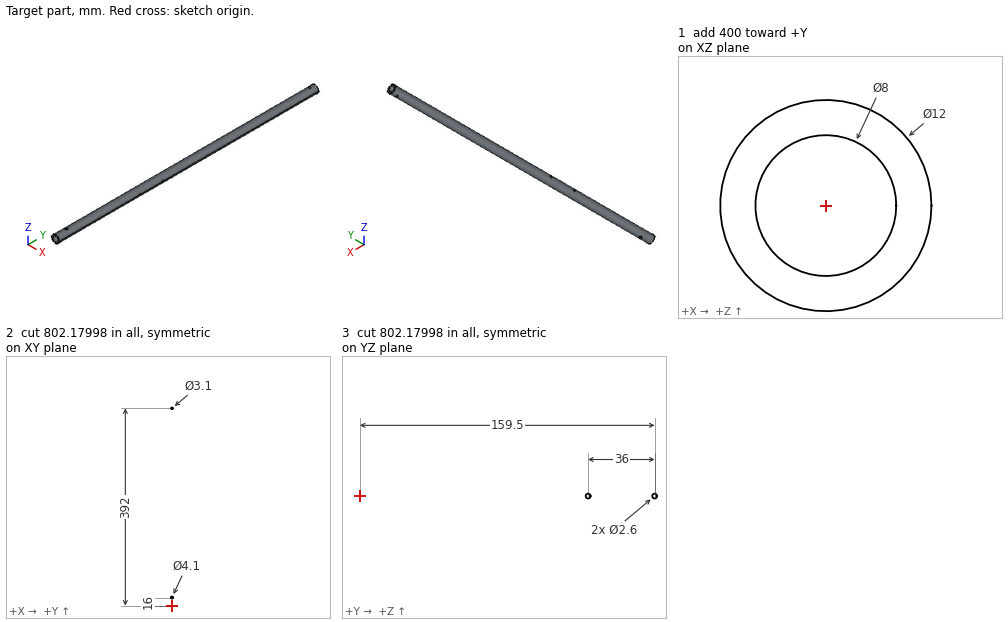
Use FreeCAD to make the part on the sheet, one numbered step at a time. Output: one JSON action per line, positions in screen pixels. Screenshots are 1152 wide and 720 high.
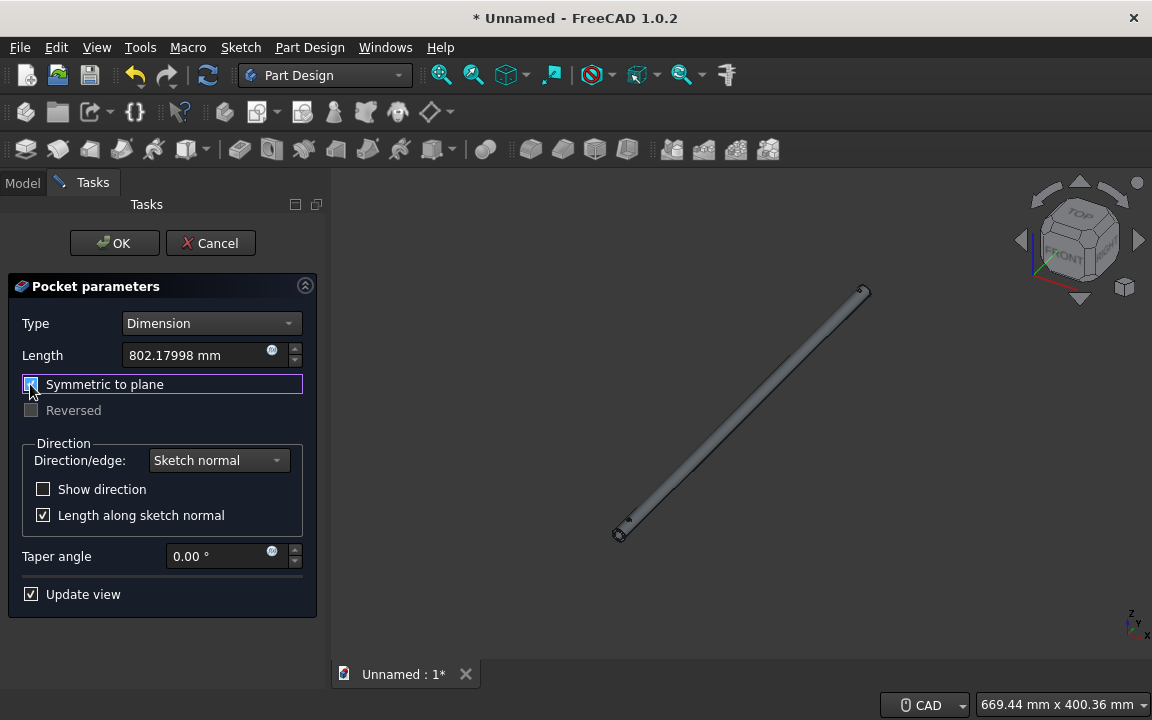
{"action": "left_click", "coordinate": [115, 243]}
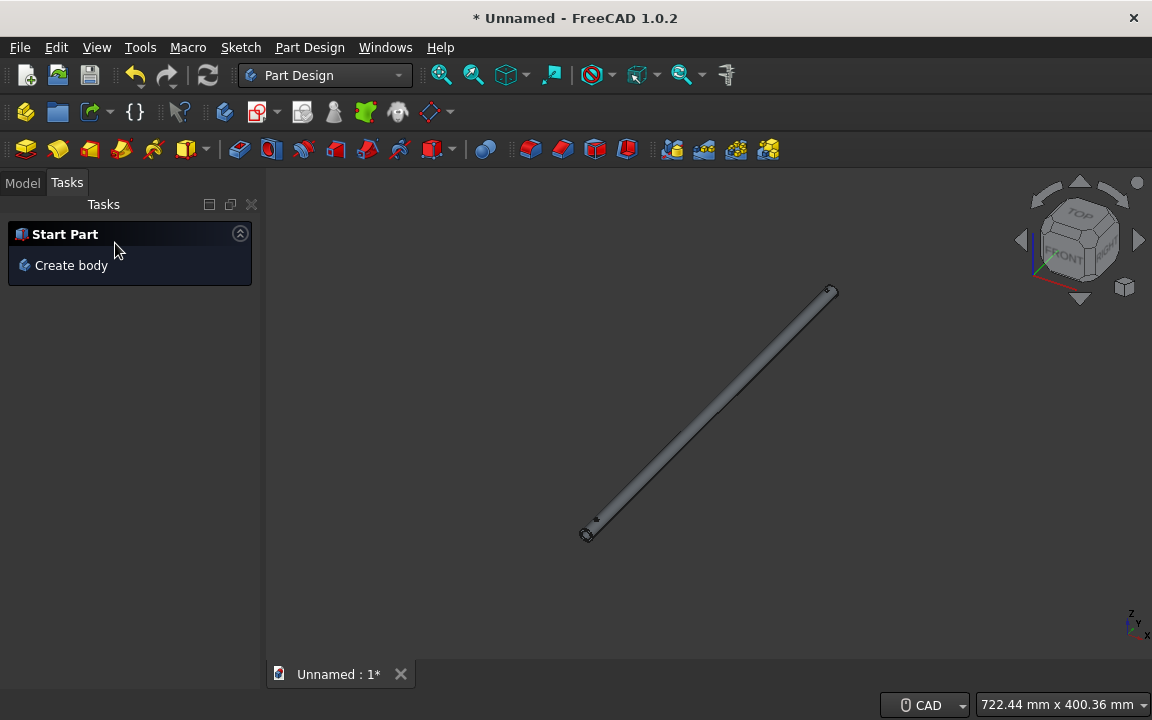
{"action": "left_click", "coordinate": [258, 112]}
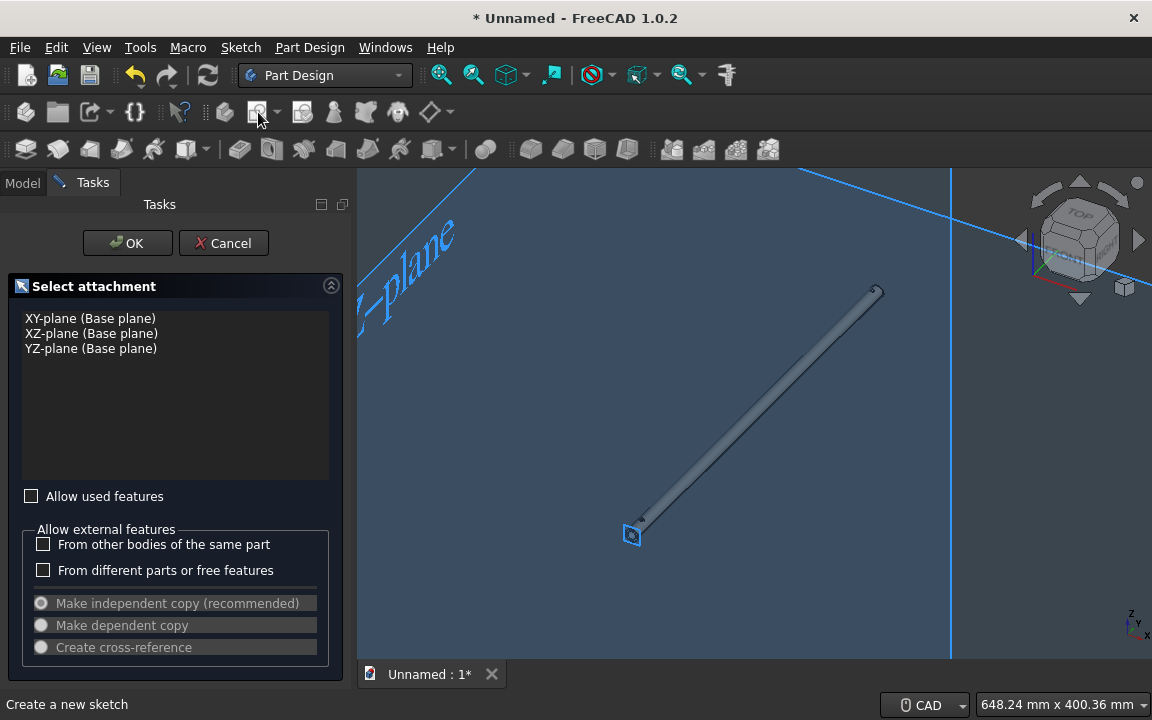
{"action": "left_click", "coordinate": [82, 348]}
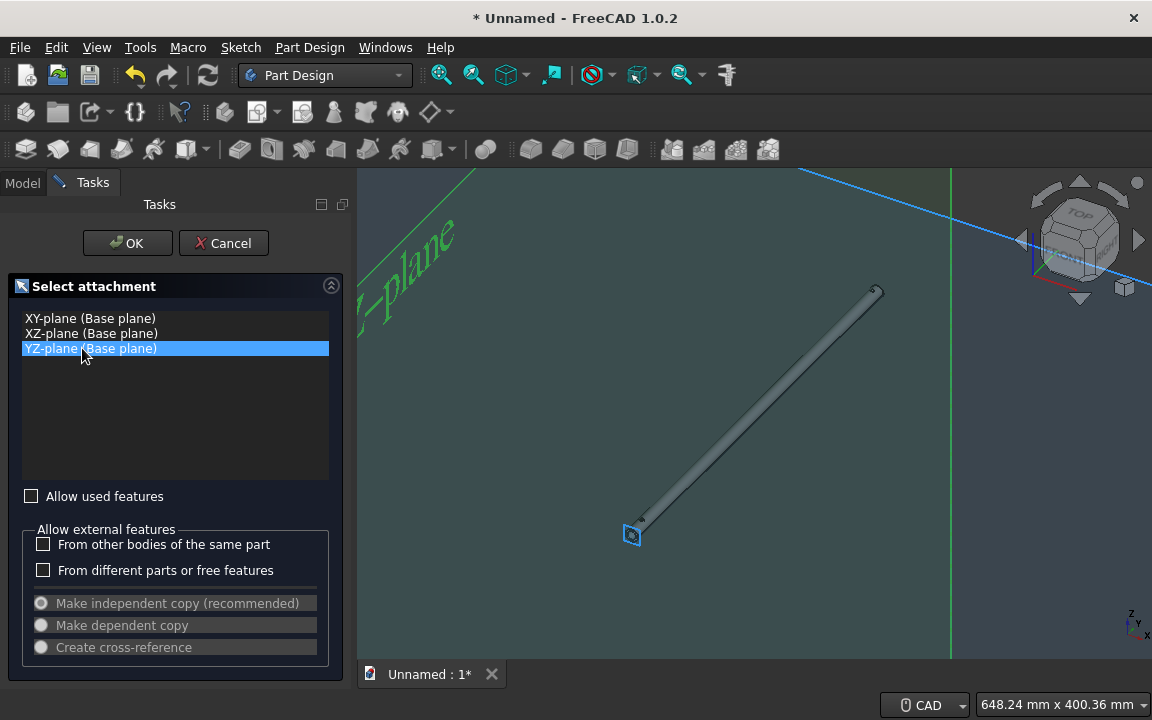
{"action": "left_click", "coordinate": [128, 243]}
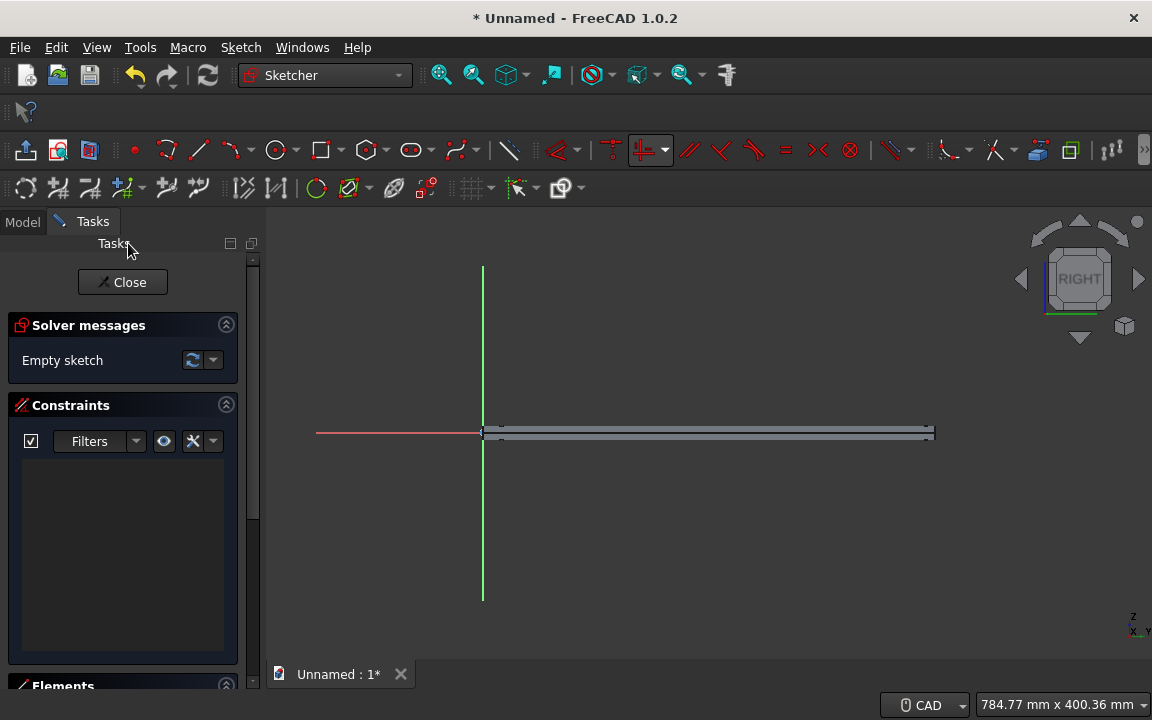
{"action": "key", "text": "q s"}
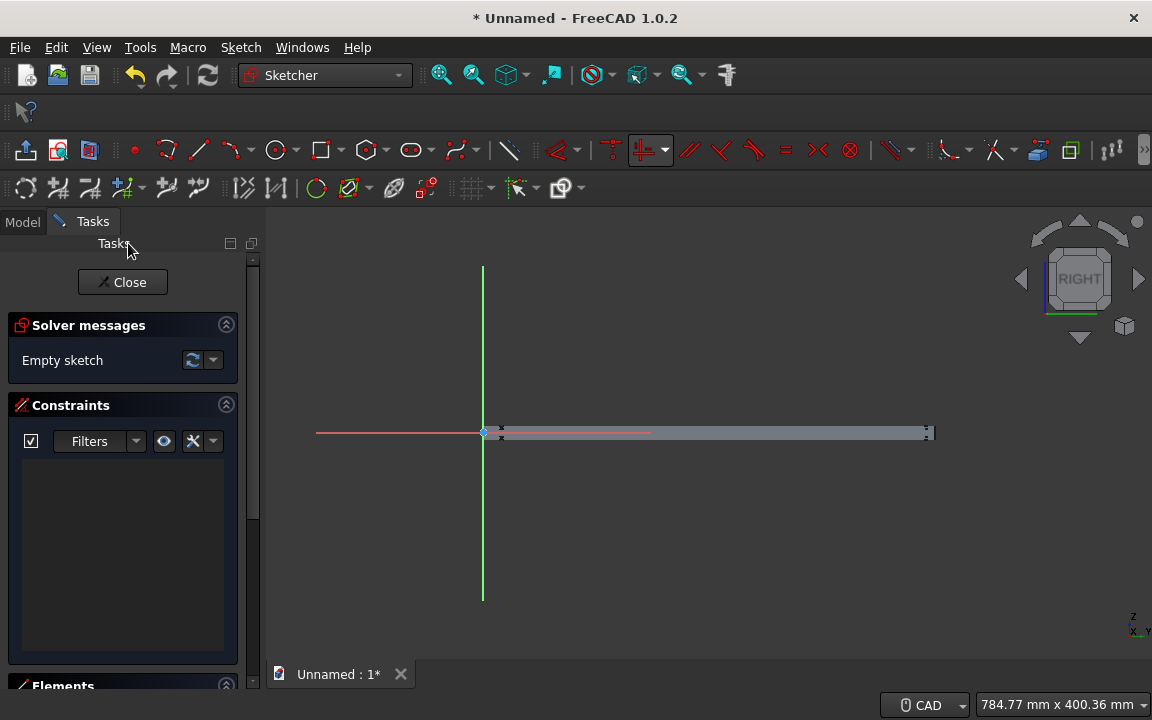
{"action": "scroll", "coordinate": [643, 433], "scroll_direction": "up", "scroll_amount": 12}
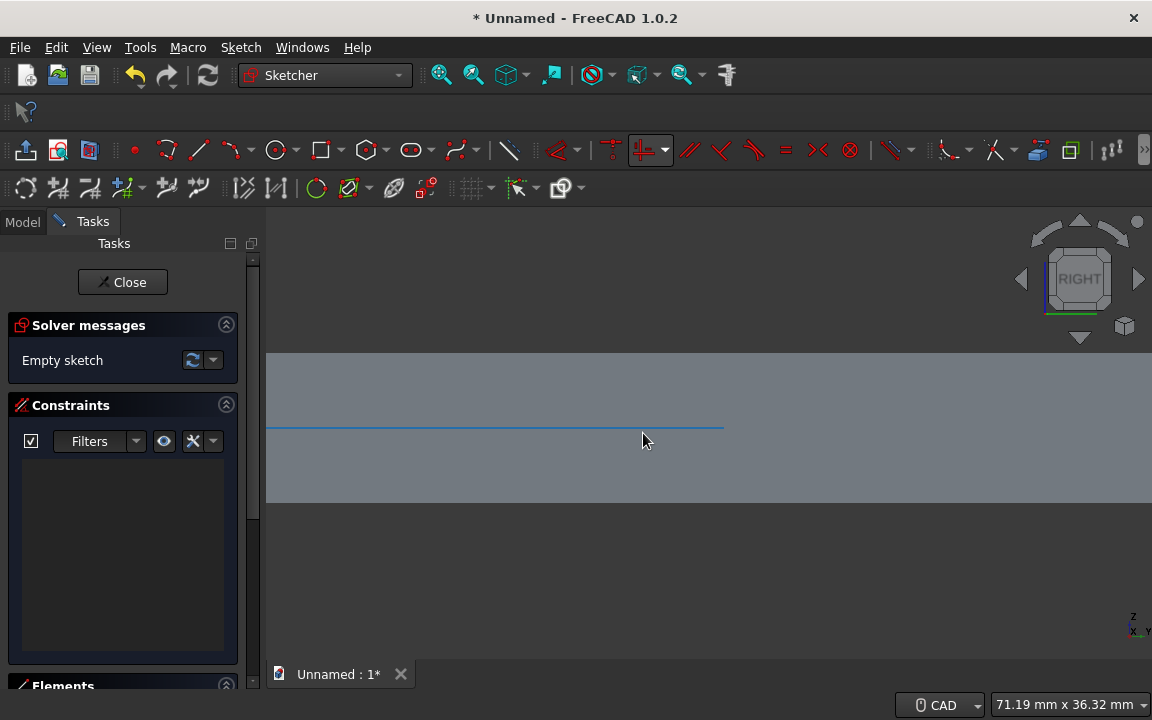
{"action": "key", "text": "g c"}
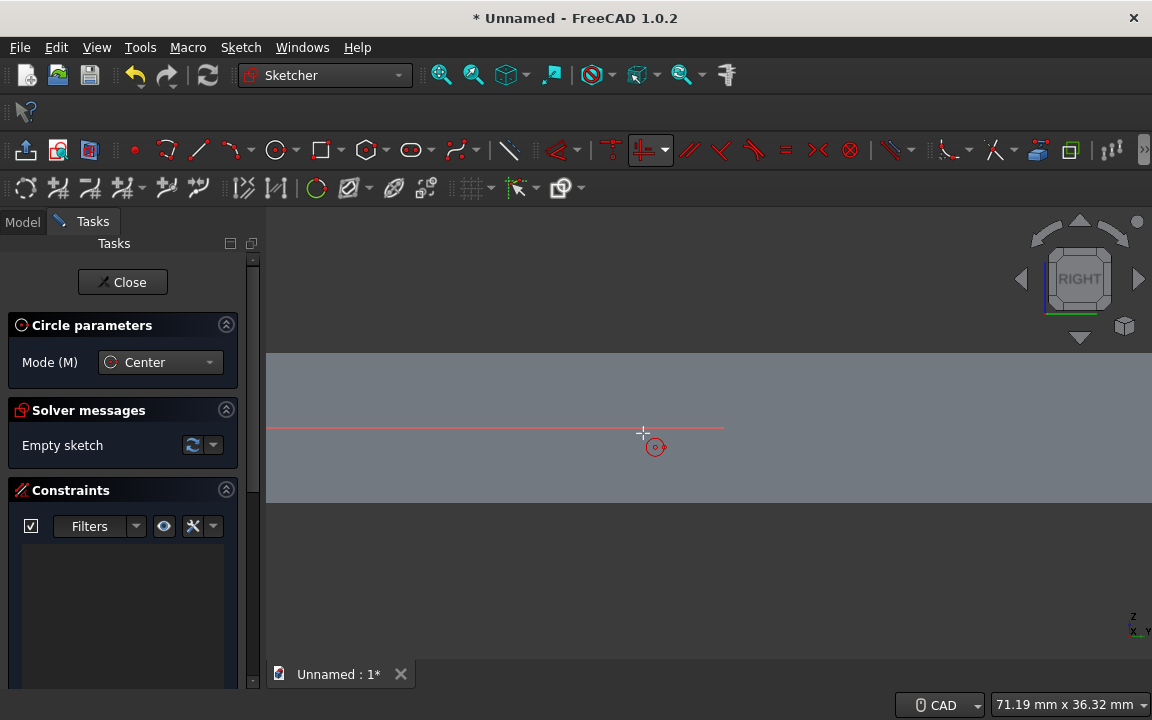
{"action": "scroll", "coordinate": [862, 428], "scroll_direction": "up", "scroll_amount": 2}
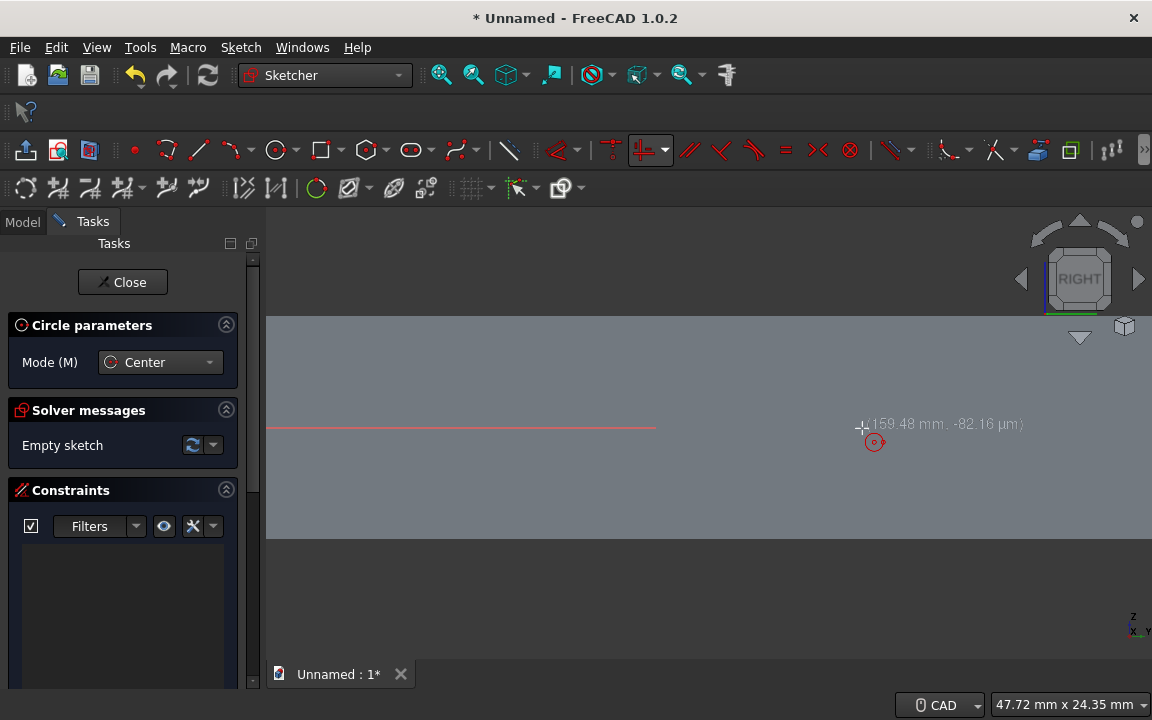
{"action": "left_click", "coordinate": [862, 428]}
{"action": "left_click", "coordinate": [879, 411]}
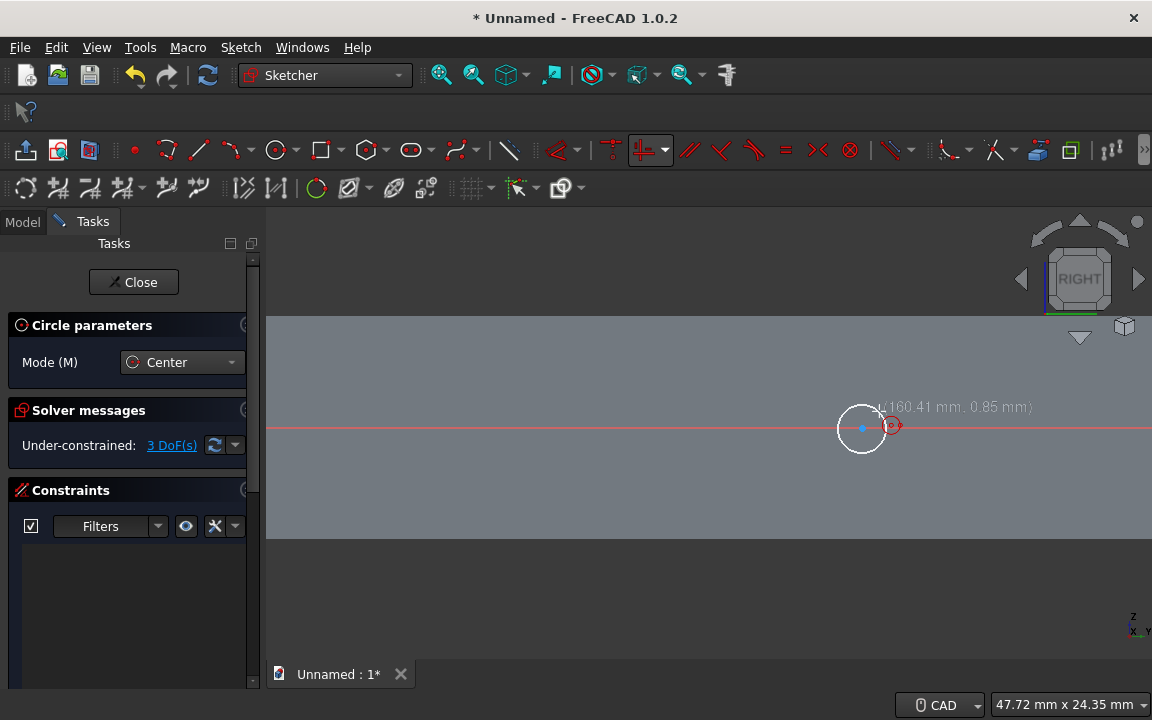
{"action": "scroll", "coordinate": [870, 444], "scroll_direction": "down", "scroll_amount": 2}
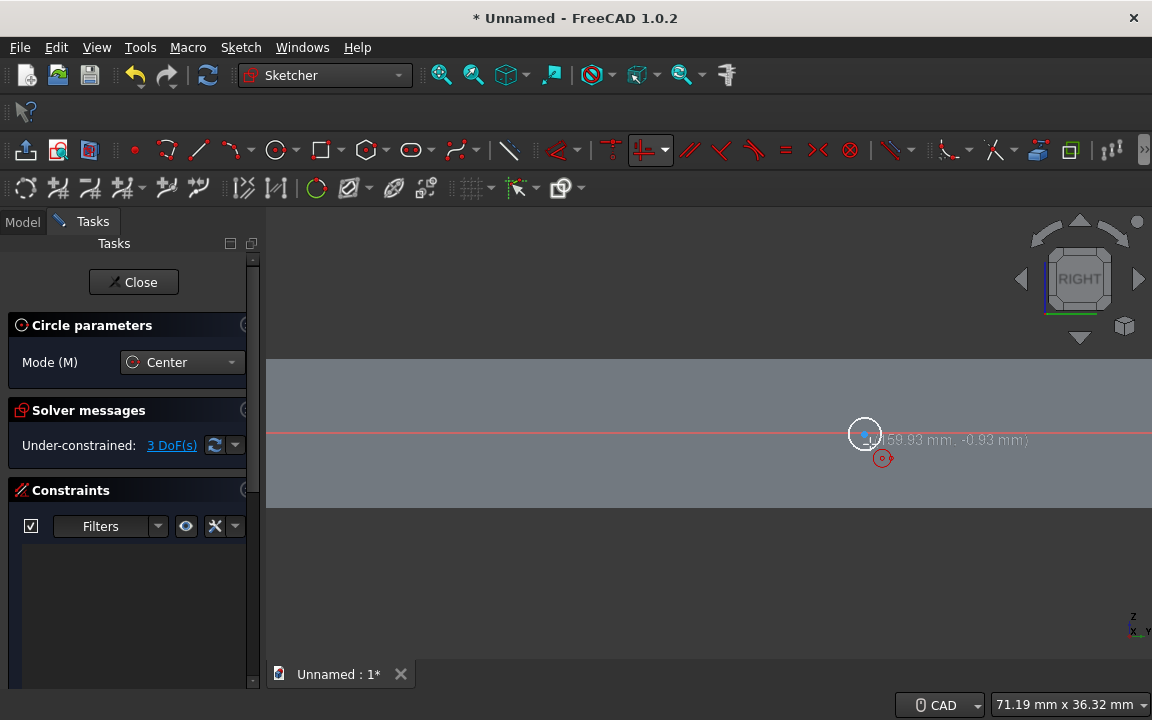
{"action": "scroll", "coordinate": [417, 433], "scroll_direction": "up", "scroll_amount": 2}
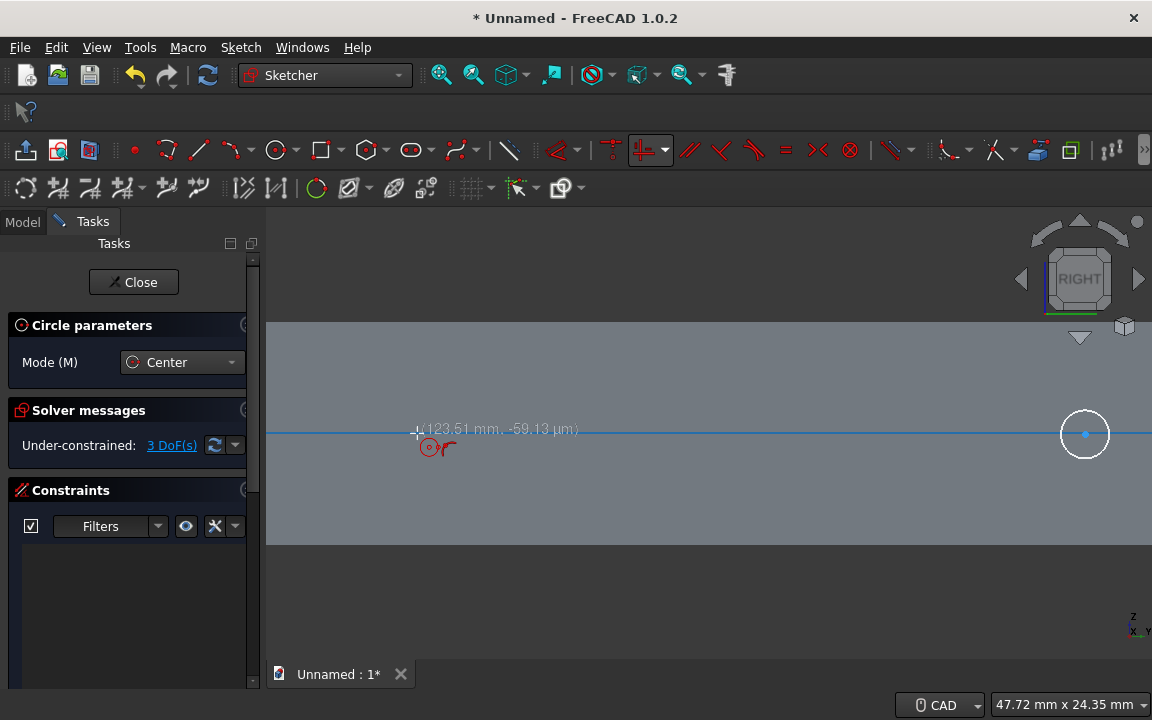
{"action": "left_click", "coordinate": [417, 433]}
{"action": "left_click", "coordinate": [434, 416]}
{"action": "key", "text": "Escape"}